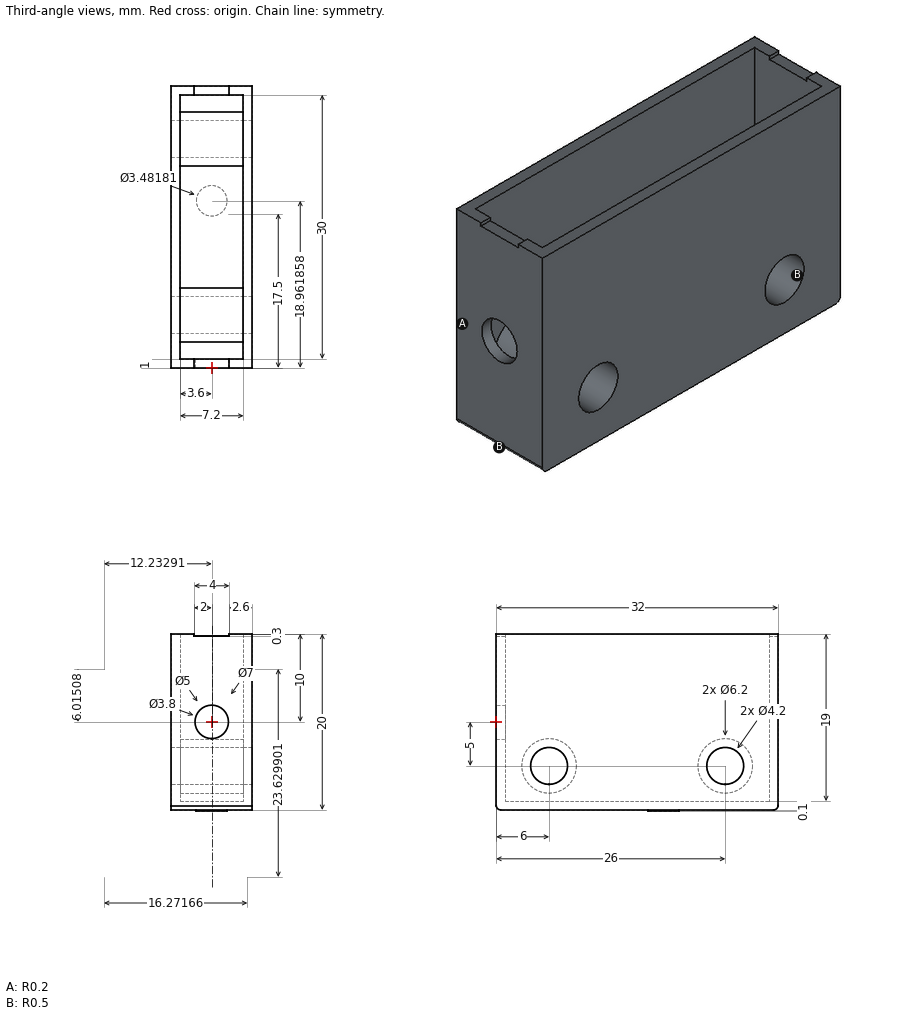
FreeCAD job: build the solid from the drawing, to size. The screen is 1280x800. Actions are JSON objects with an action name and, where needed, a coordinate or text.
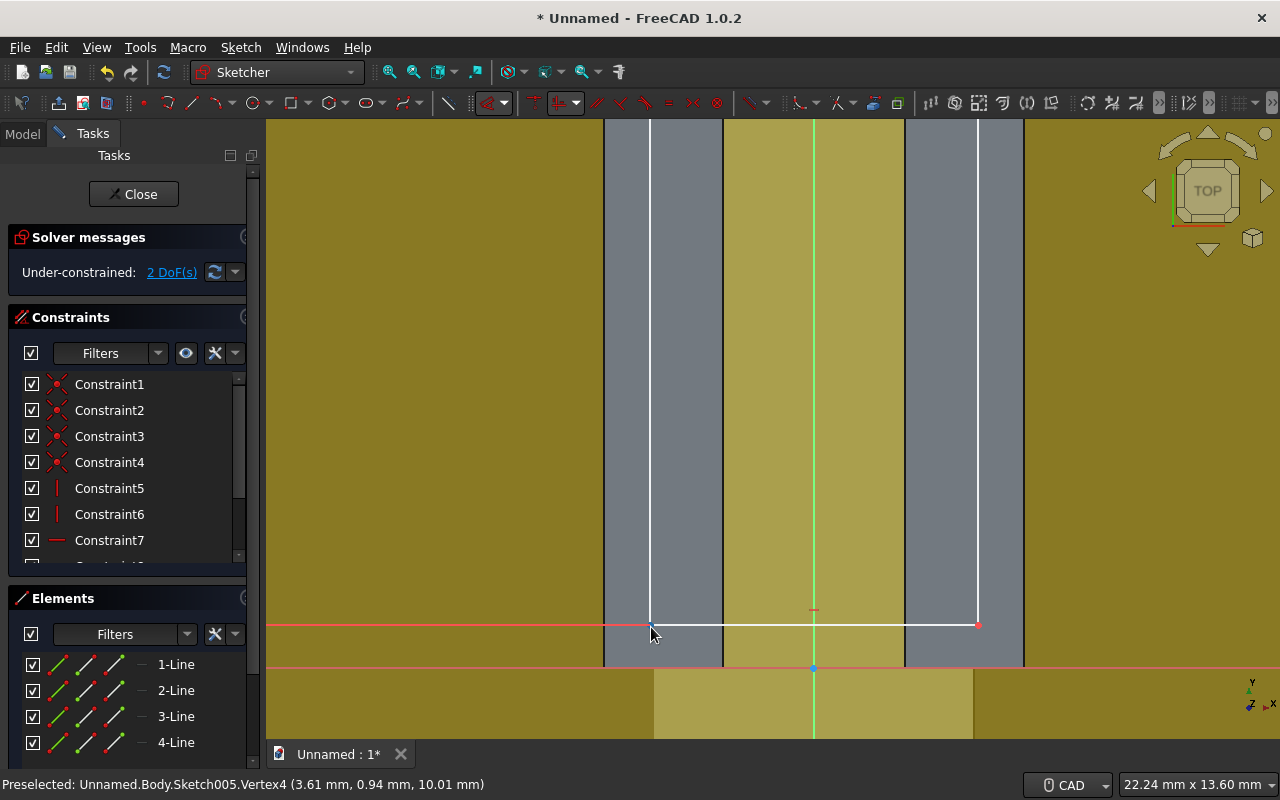
{"action": "left_click", "coordinate": [650, 625]}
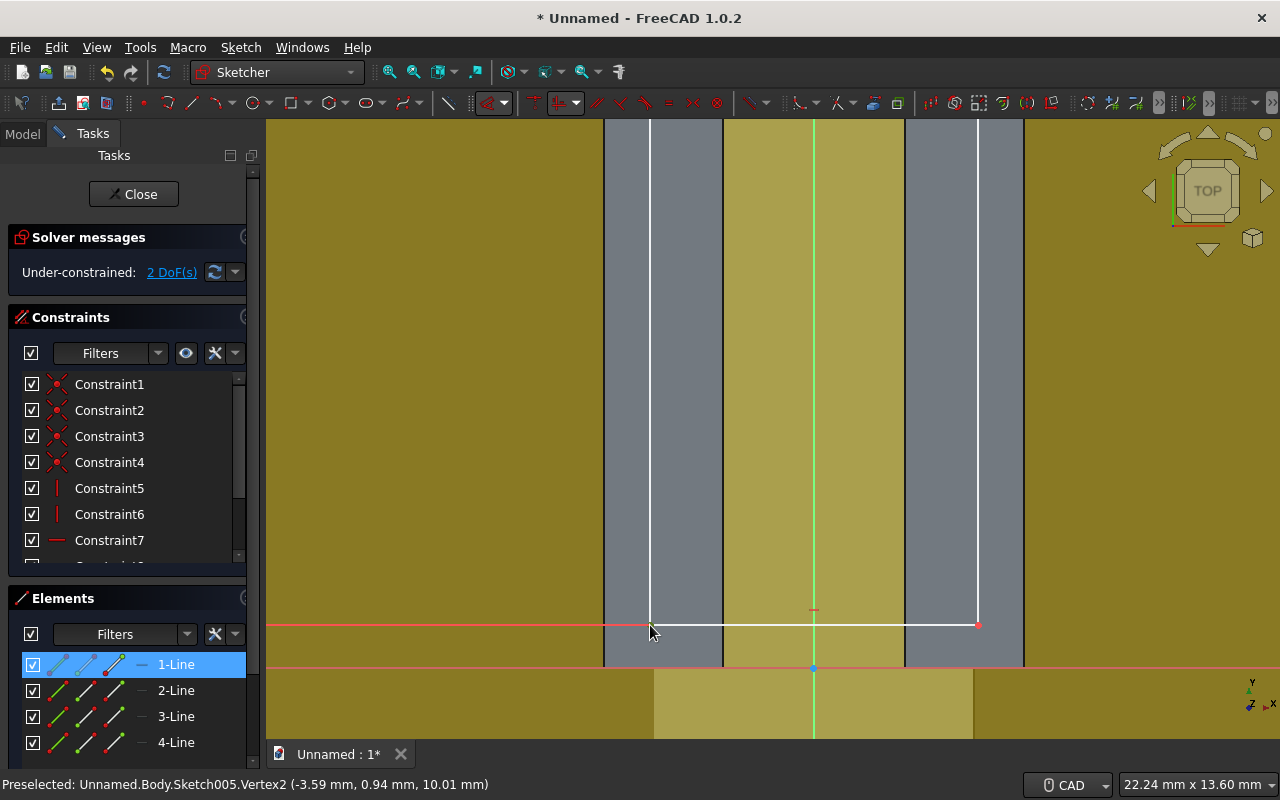
{"action": "left_click", "coordinate": [506, 104]}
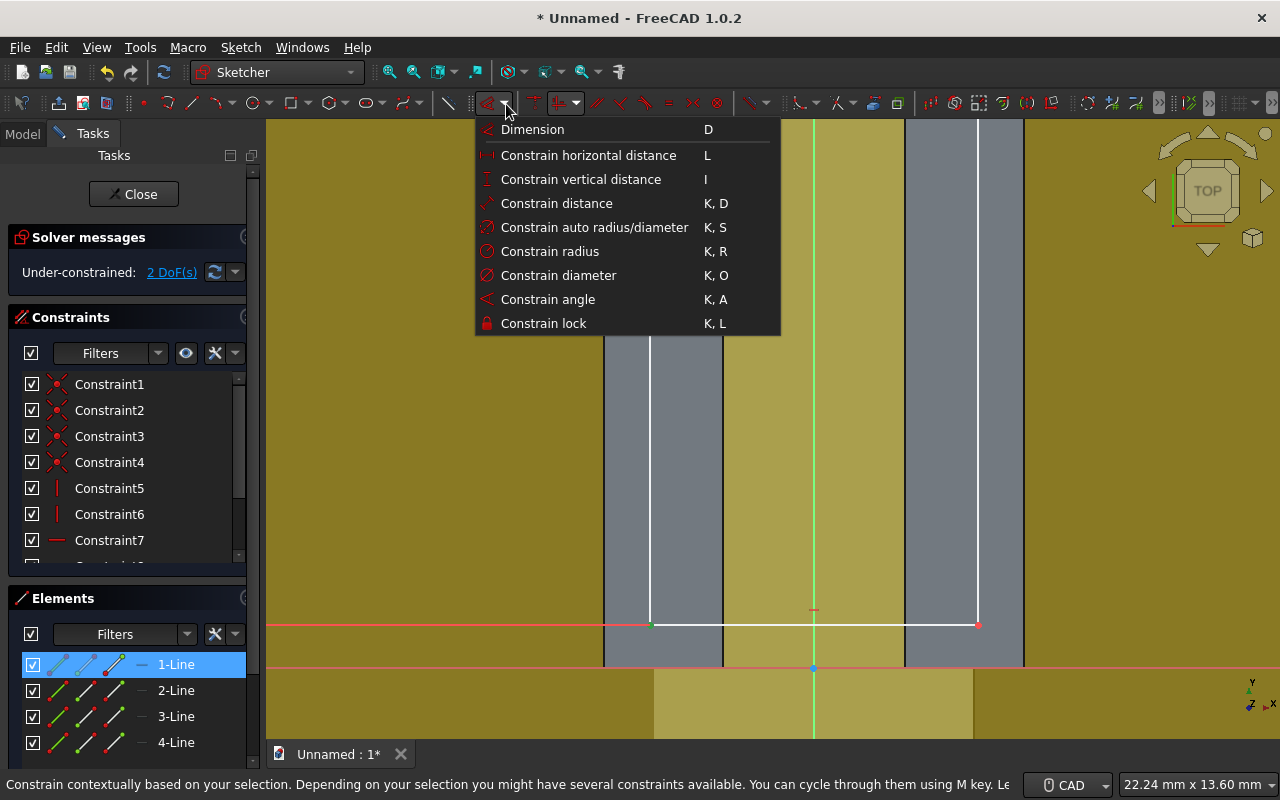
{"action": "left_click", "coordinate": [628, 179]}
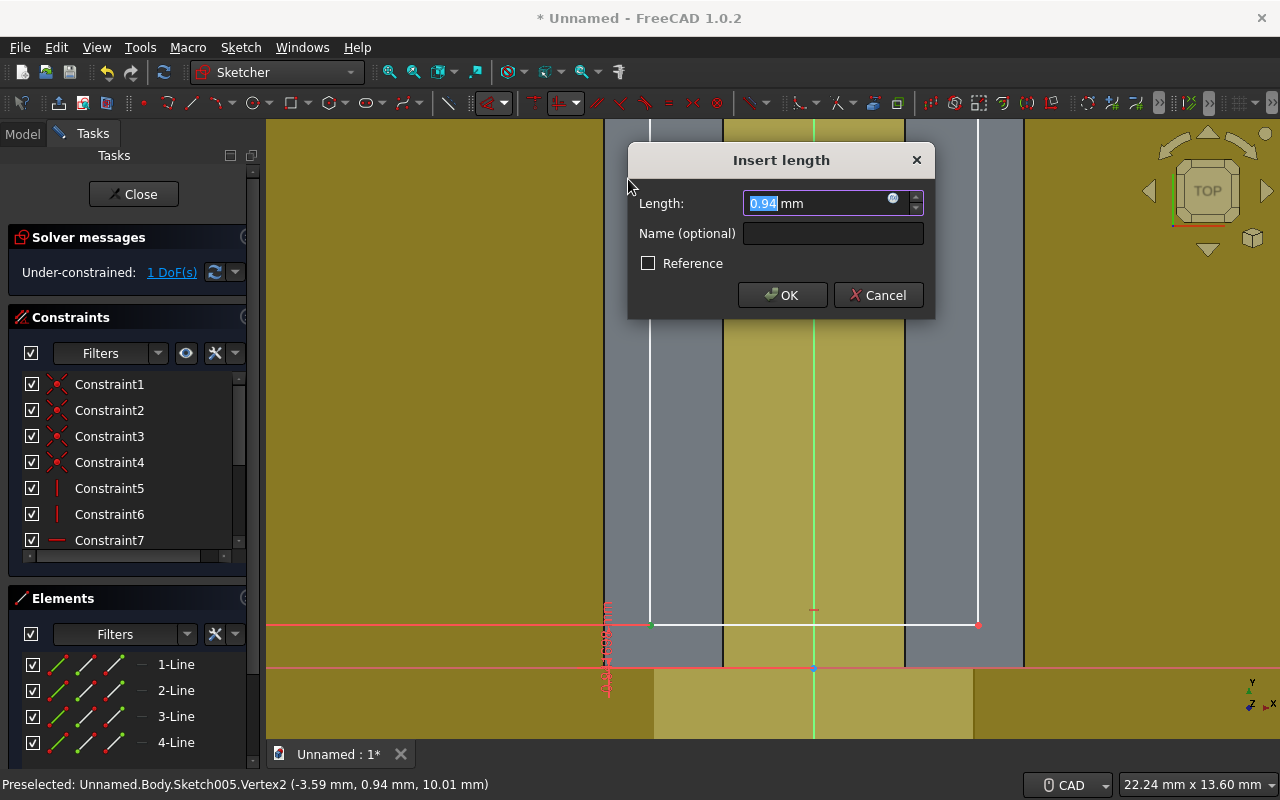
{"action": "type", "text": "1"}
{"action": "key", "text": "Return"}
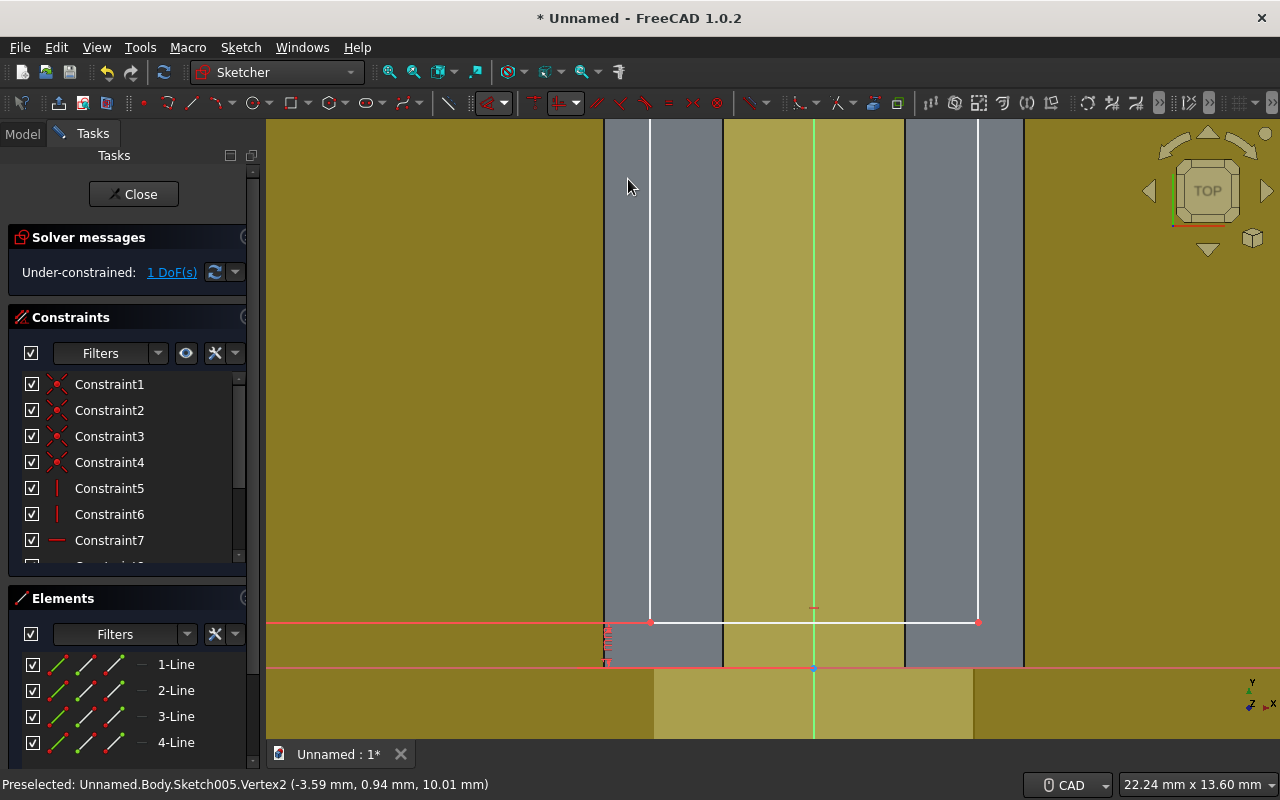
{"action": "scroll", "coordinate": [657, 631], "scroll_direction": "down", "scroll_amount": 6}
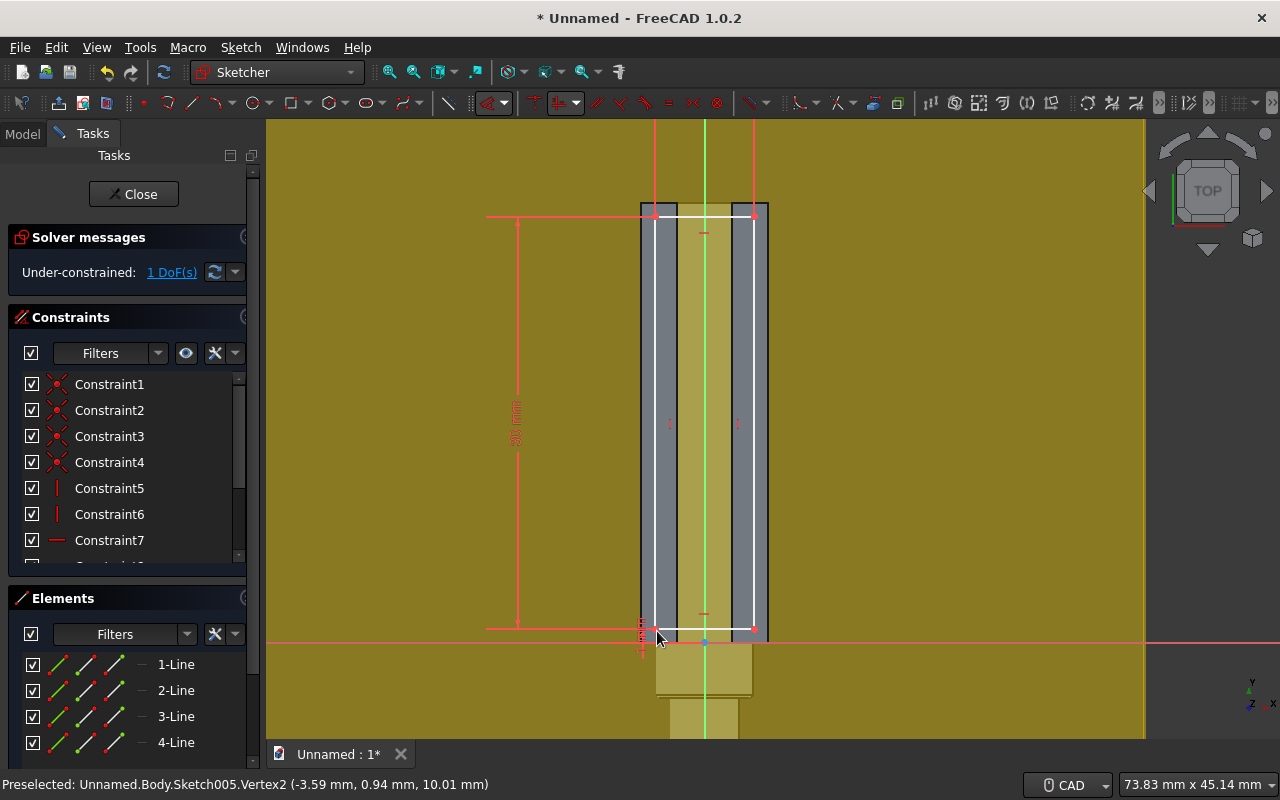
{"action": "left_click", "coordinate": [655, 217]}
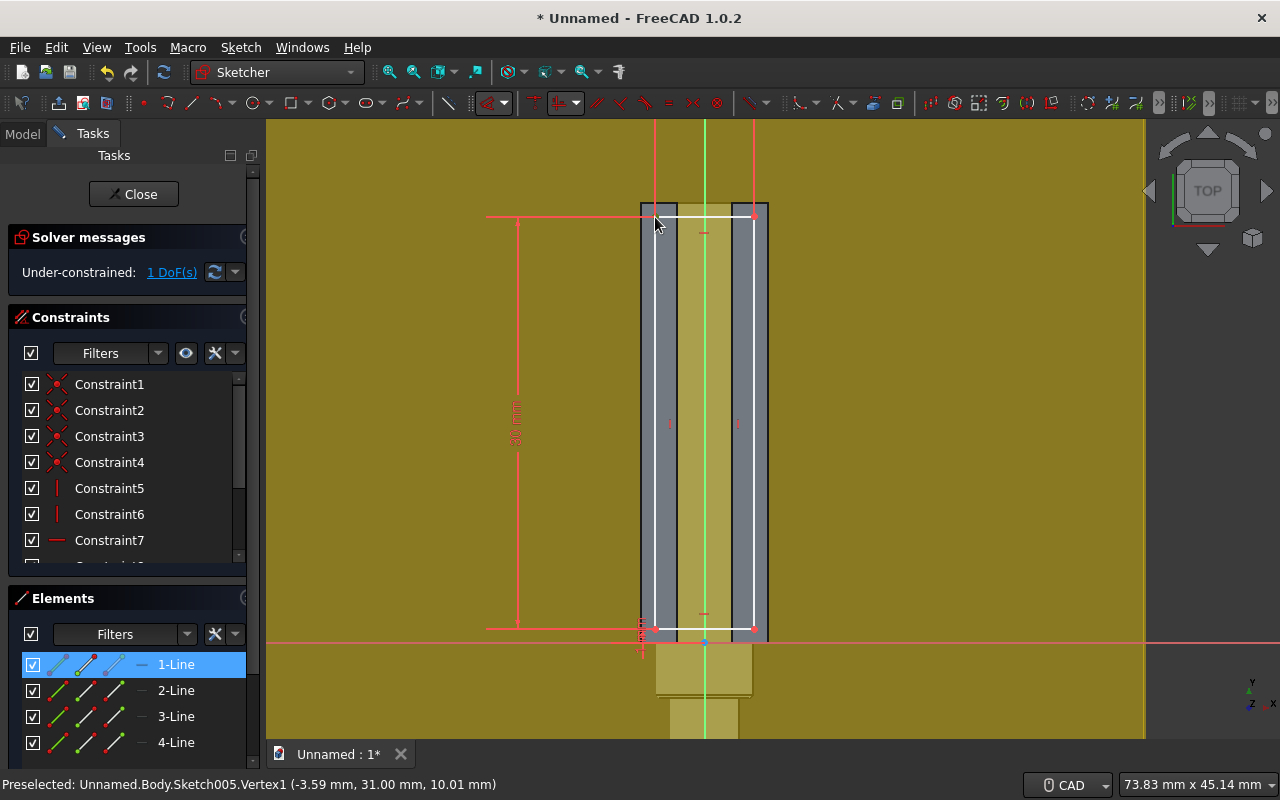
{"action": "key", "text": "l"}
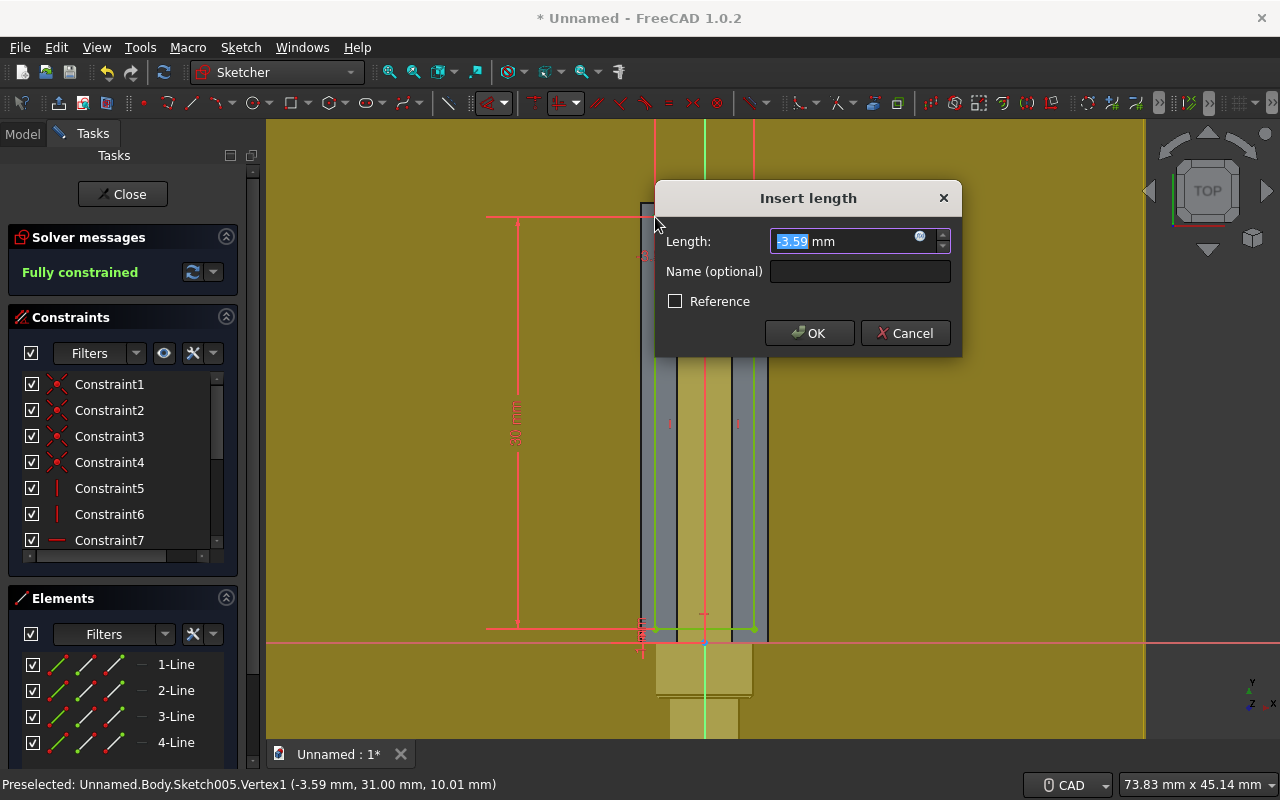
{"action": "type", "text": "-3.6"}
{"action": "key", "text": "Return"}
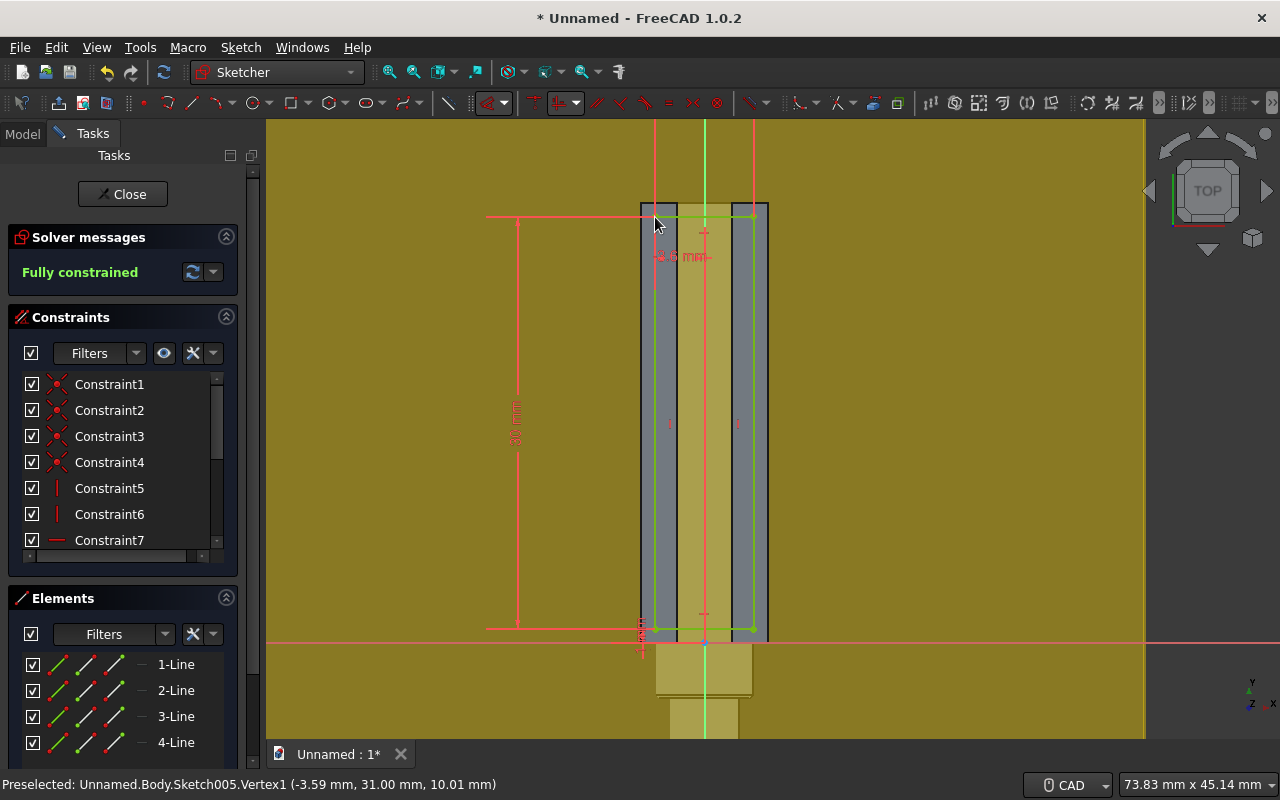
{"action": "left_click", "coordinate": [123, 194]}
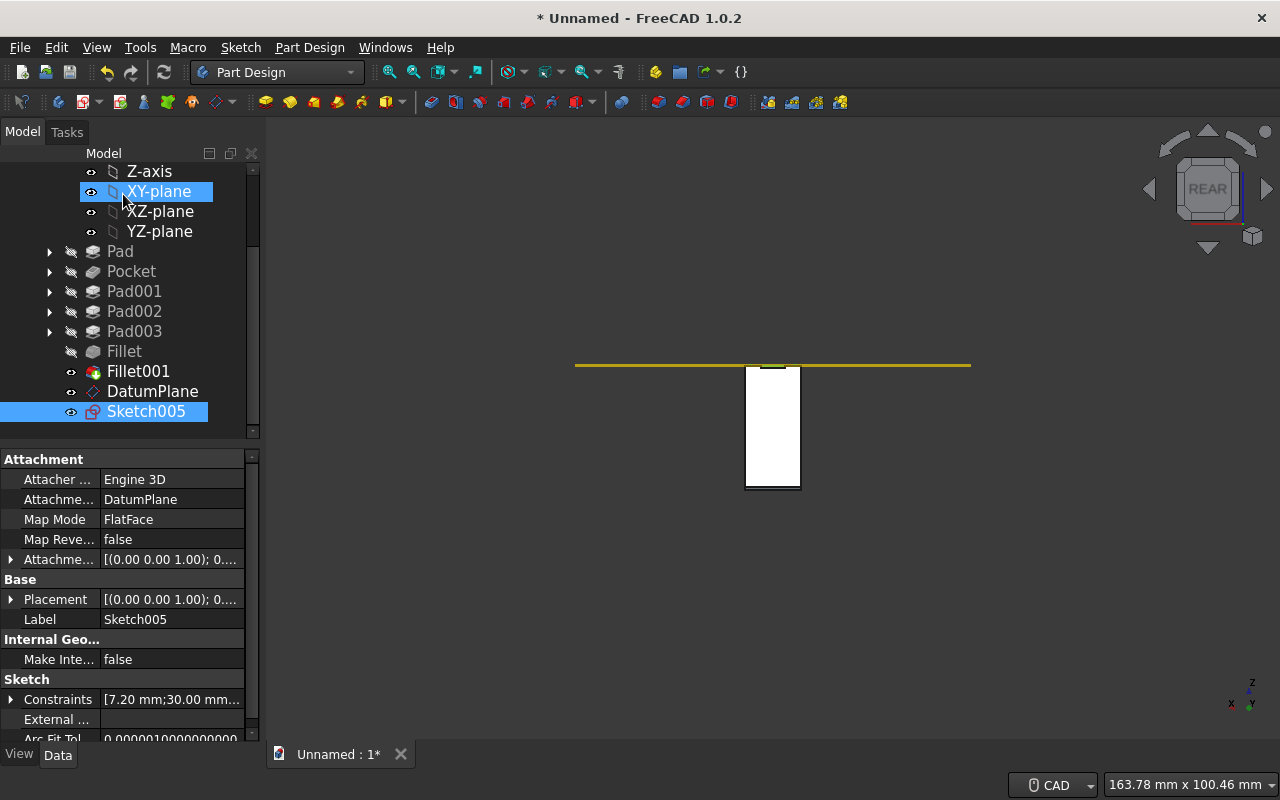
{"action": "left_click", "coordinate": [432, 102]}